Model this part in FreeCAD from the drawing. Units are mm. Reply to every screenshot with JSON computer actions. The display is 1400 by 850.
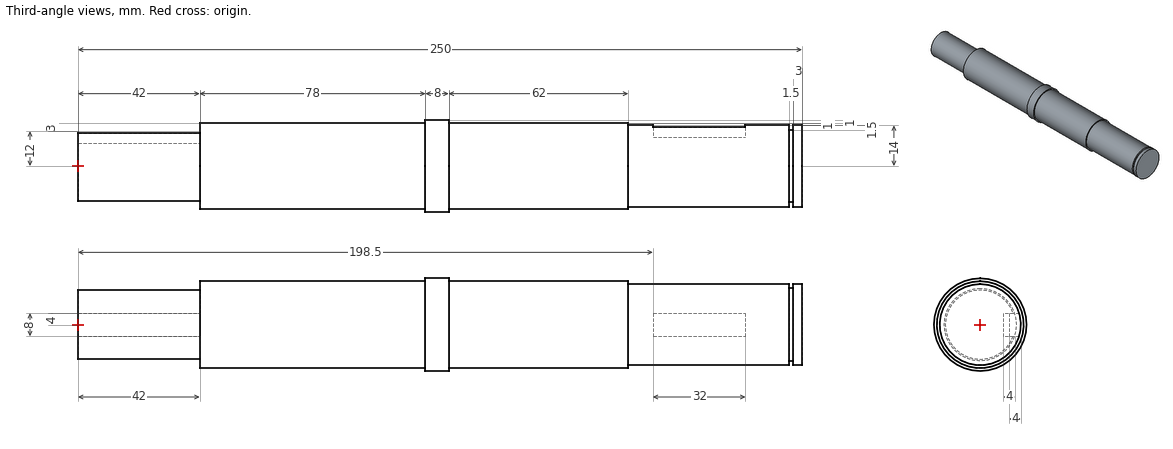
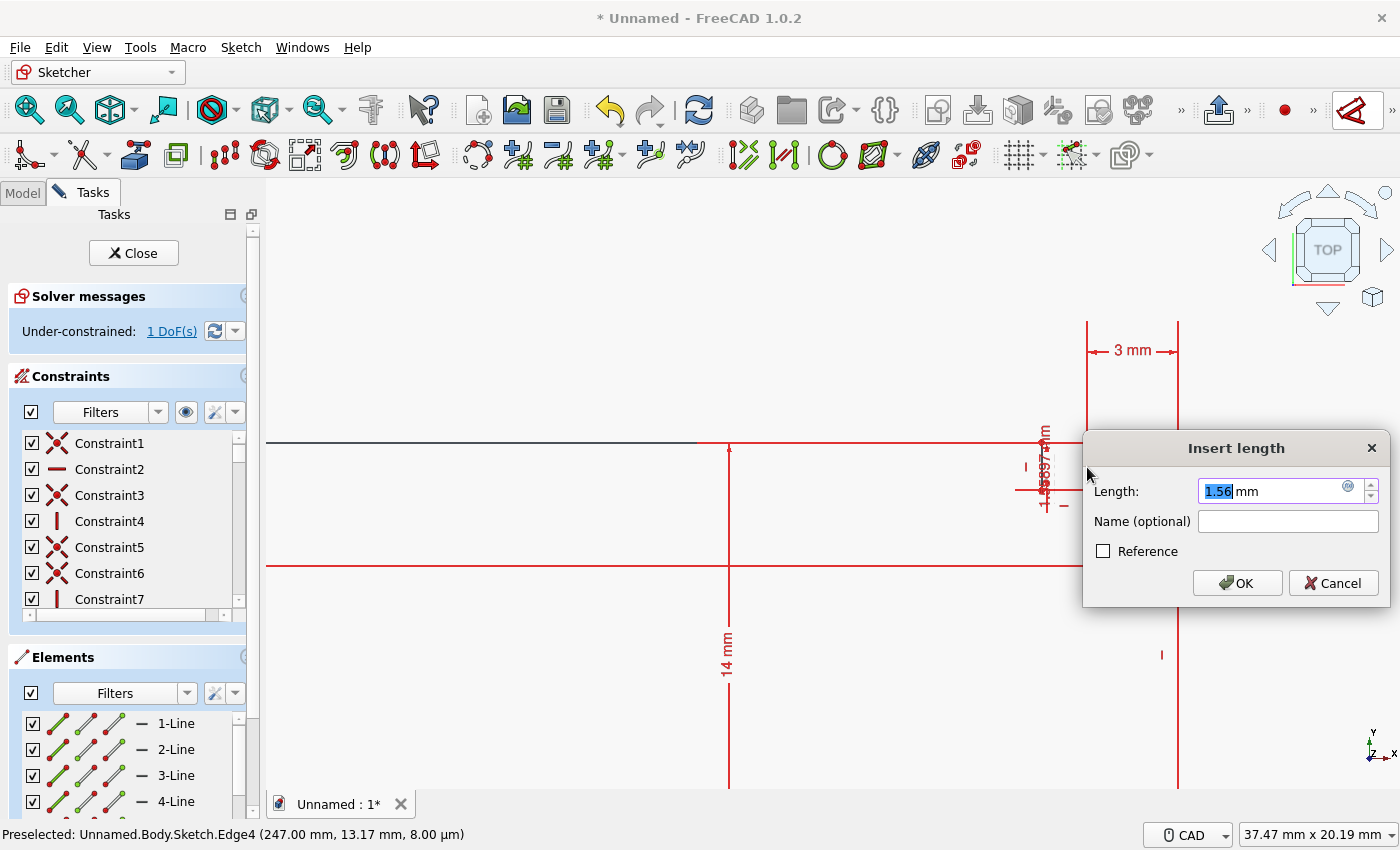
{"action": "type", "text": "1.5"}
{"action": "key", "text": "Return"}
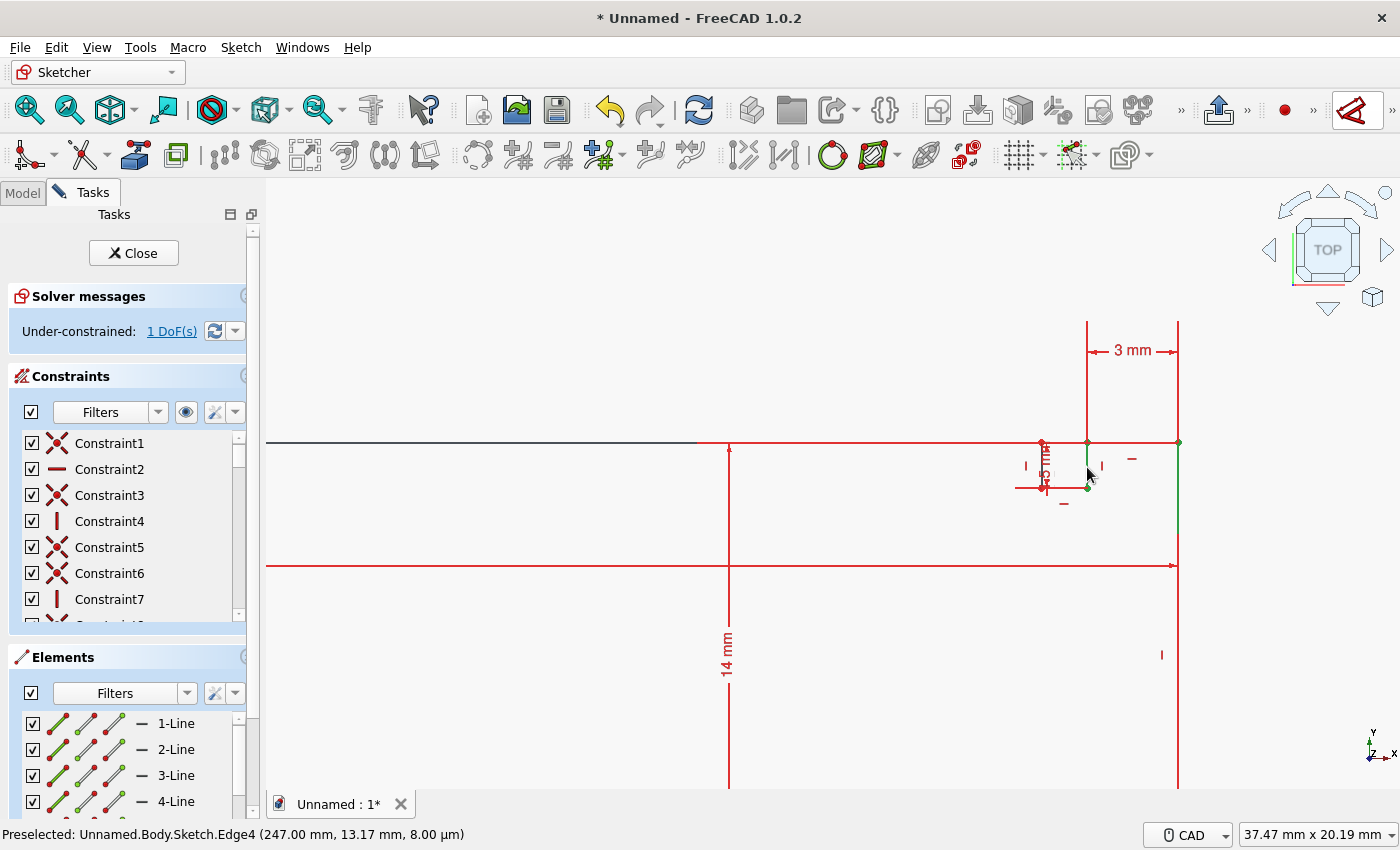
{"action": "left_click", "coordinate": [1074, 488]}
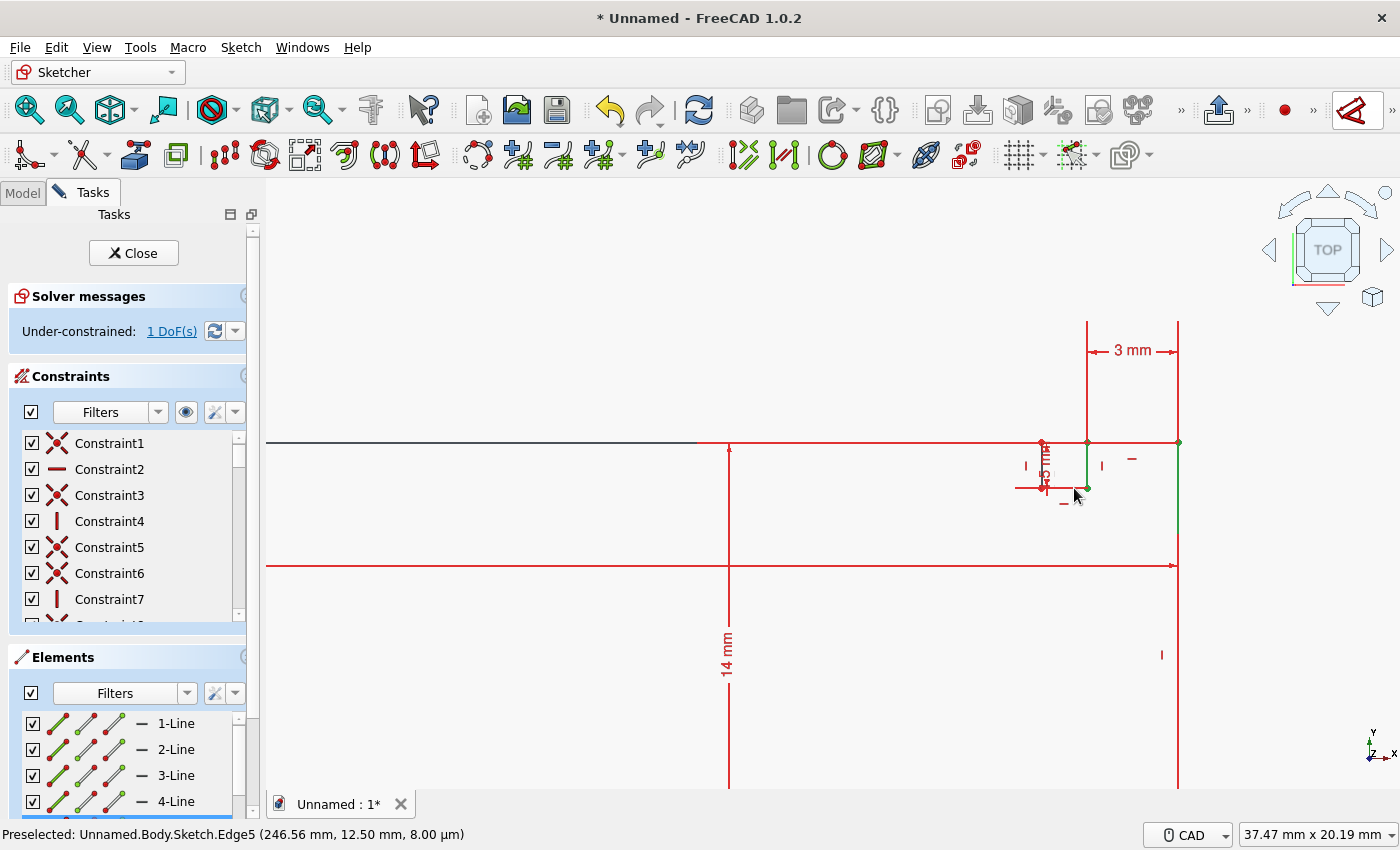
{"action": "key", "text": "l"}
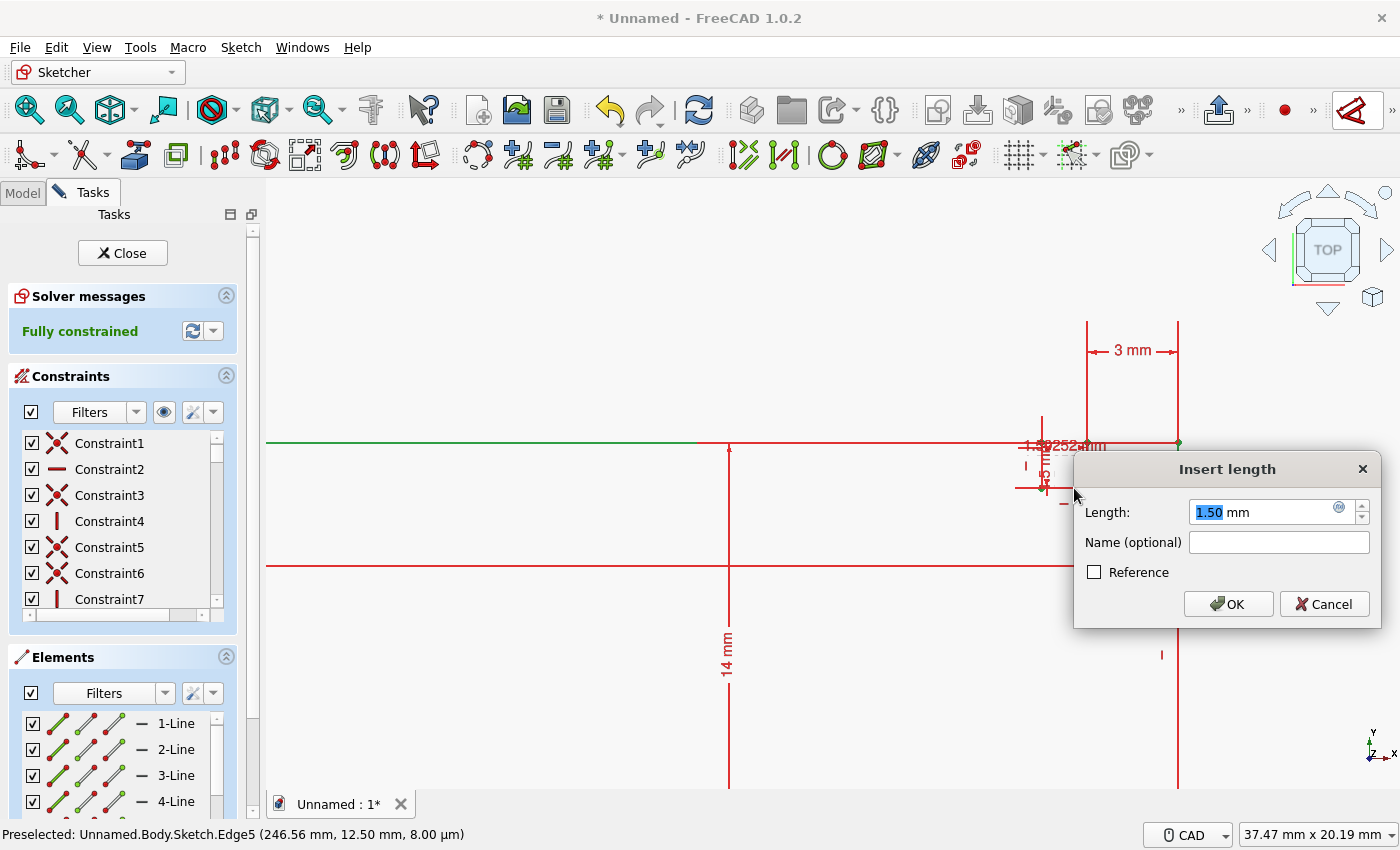
{"action": "type", "text": "1.5"}
{"action": "key", "text": "Return"}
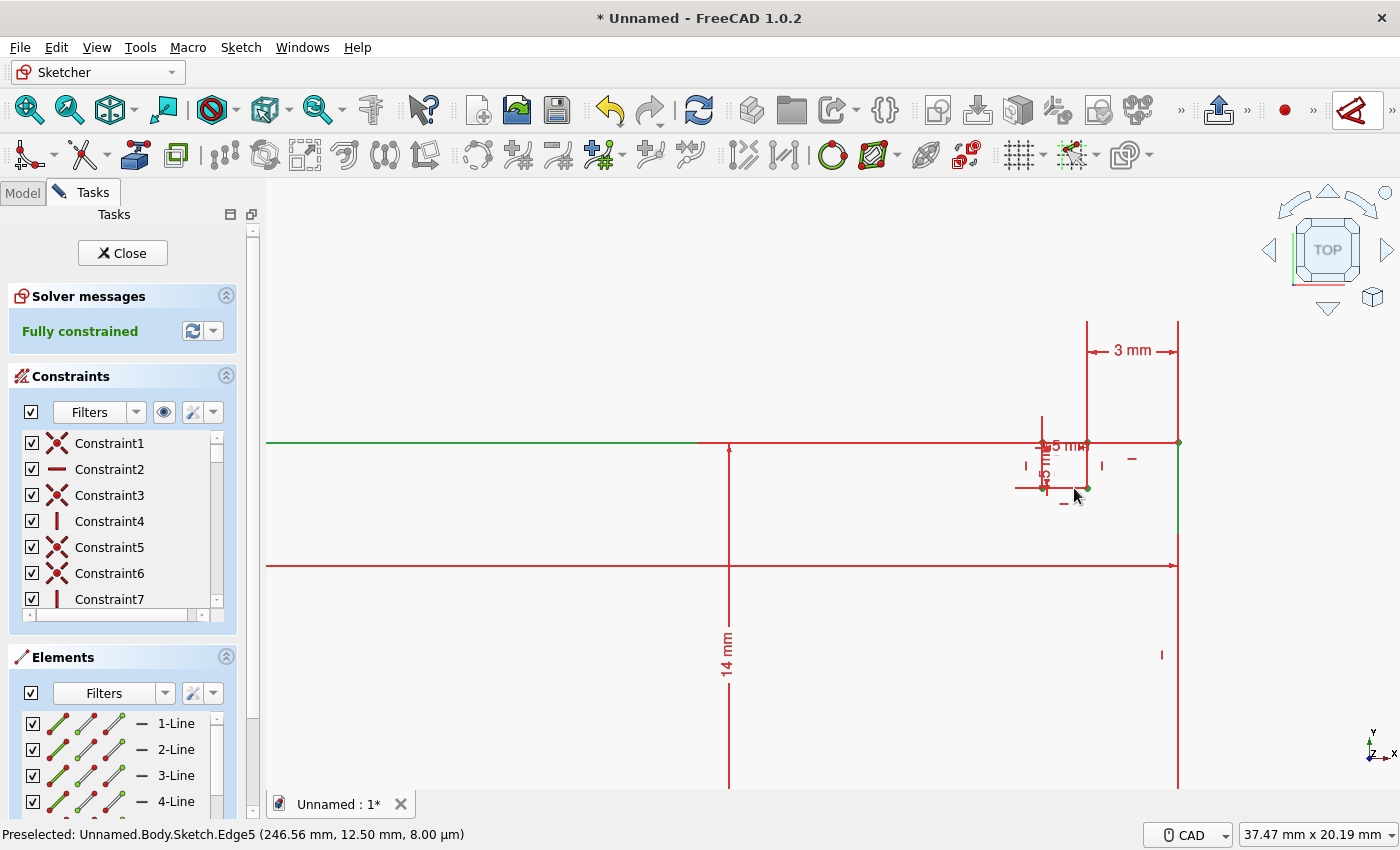
{"action": "left_click", "coordinate": [123, 253]}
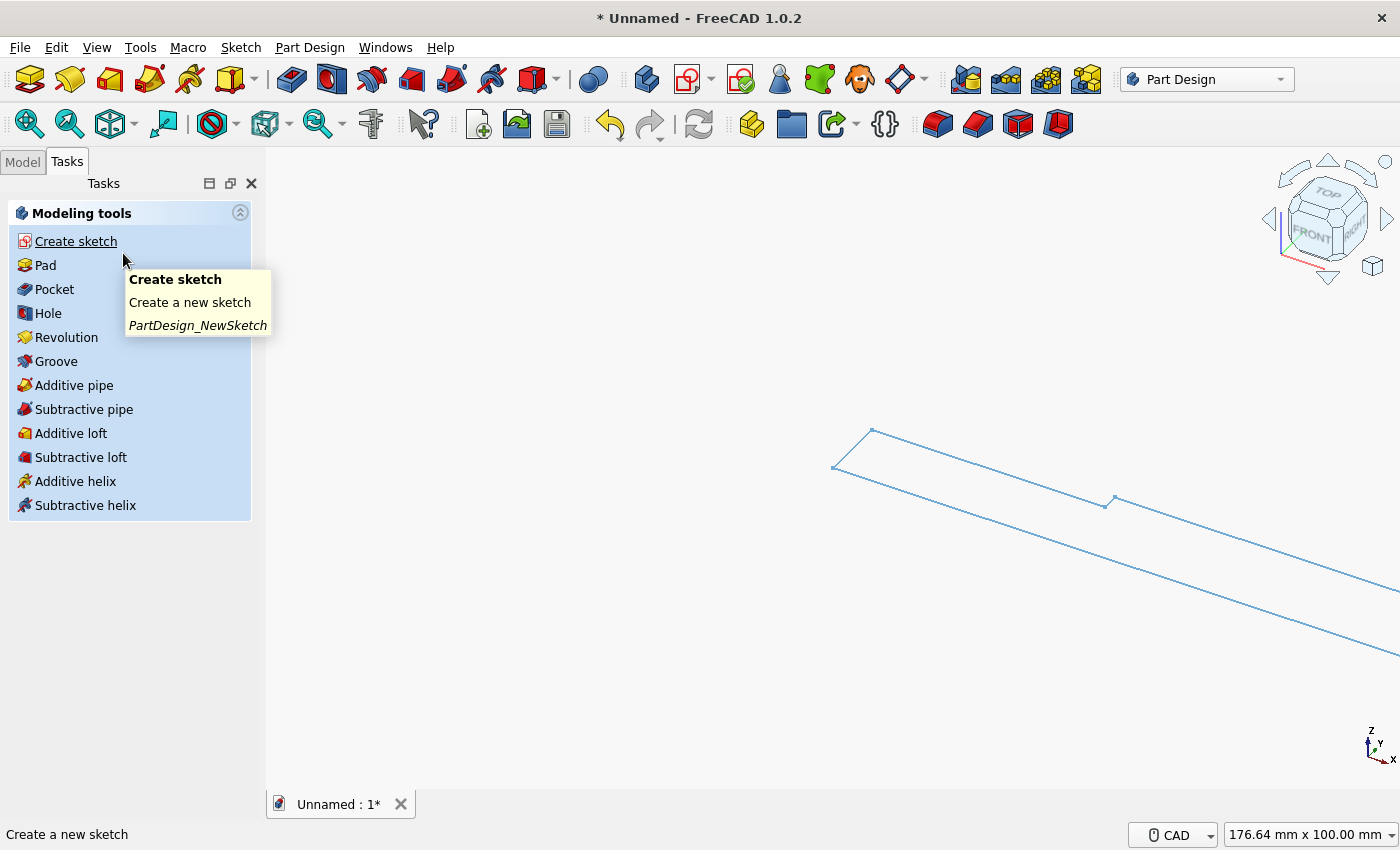
{"action": "left_click", "coordinate": [70, 80]}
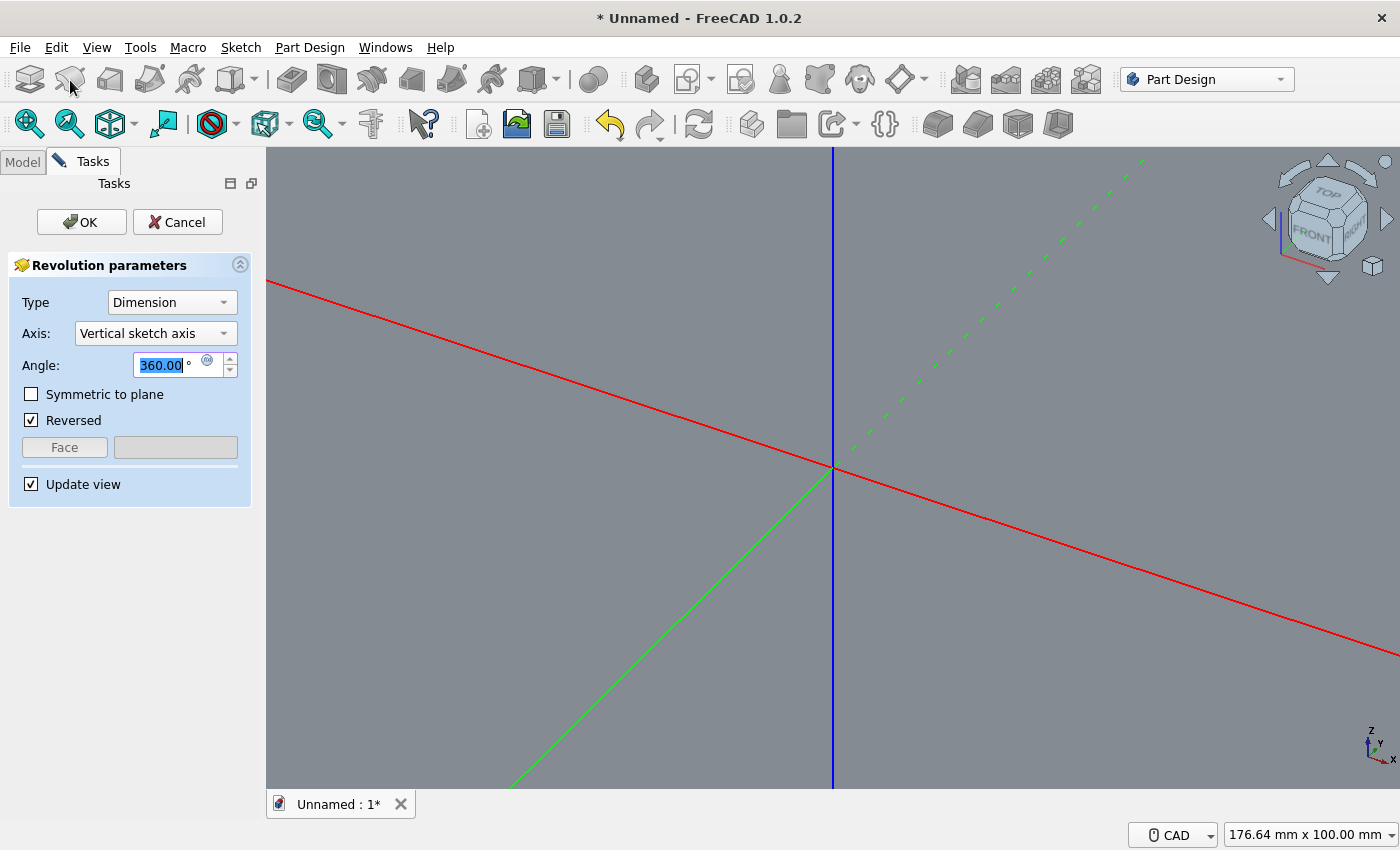
{"action": "left_click", "coordinate": [156, 334]}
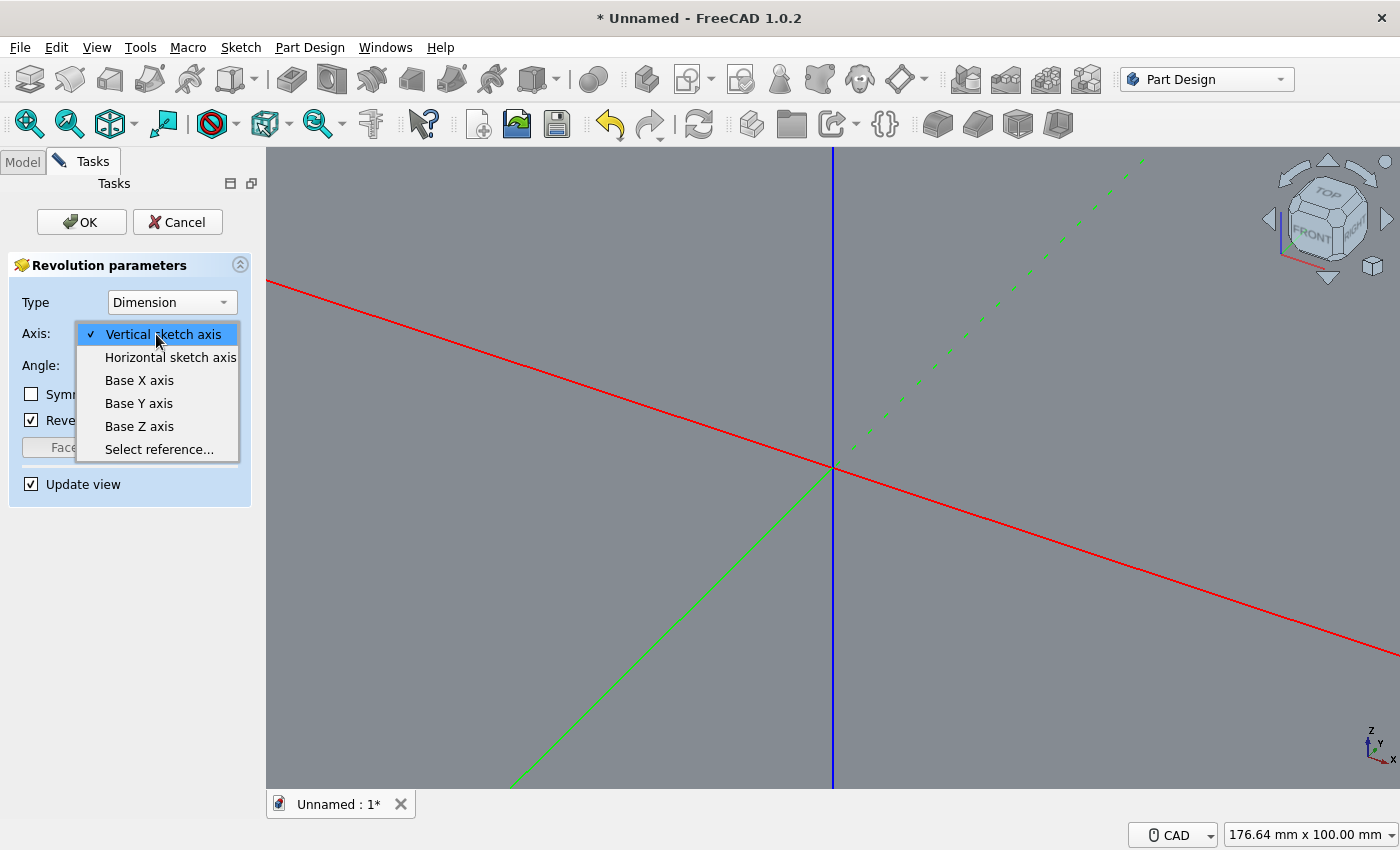
{"action": "left_click", "coordinate": [156, 358]}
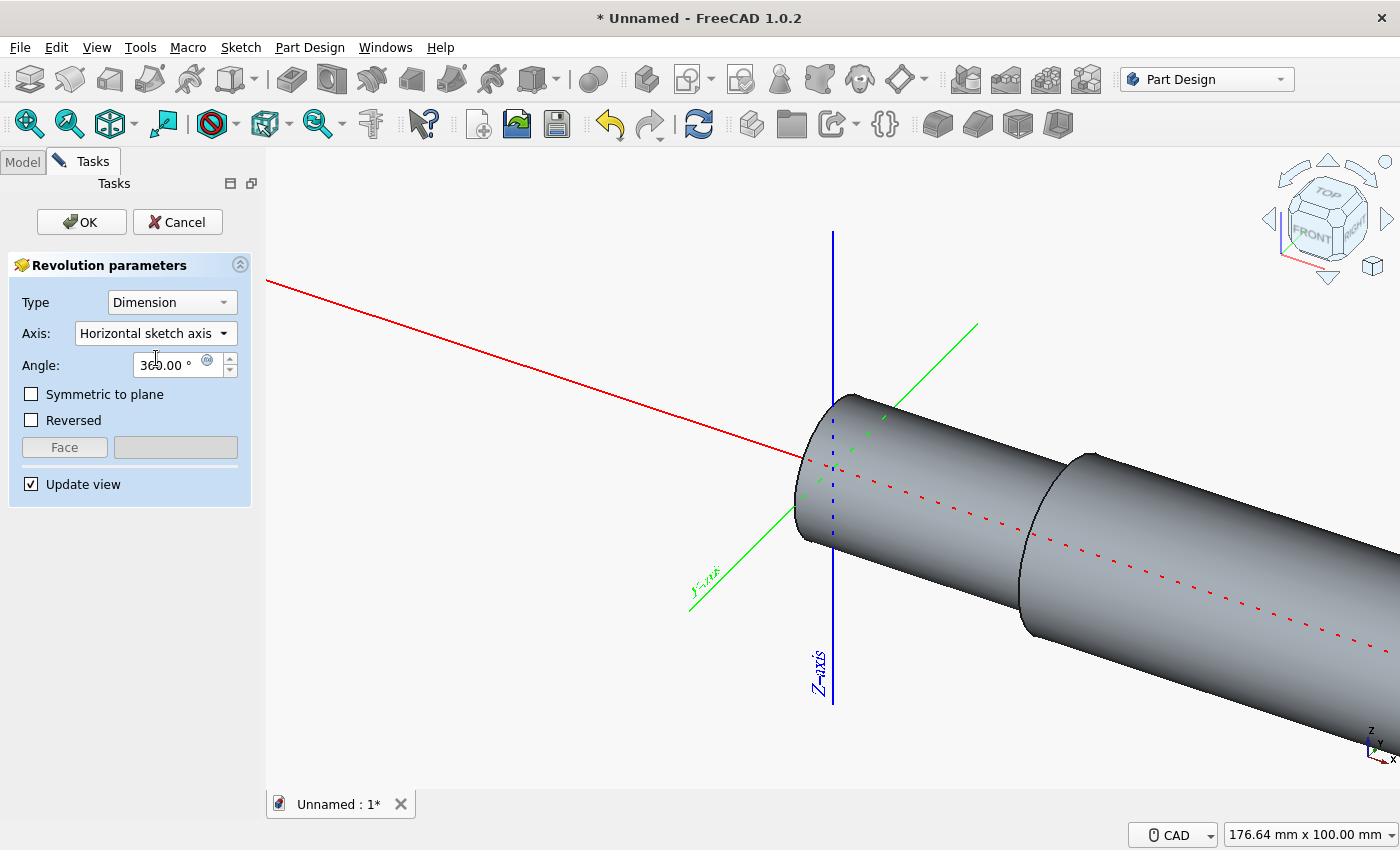
{"action": "left_click", "coordinate": [82, 222]}